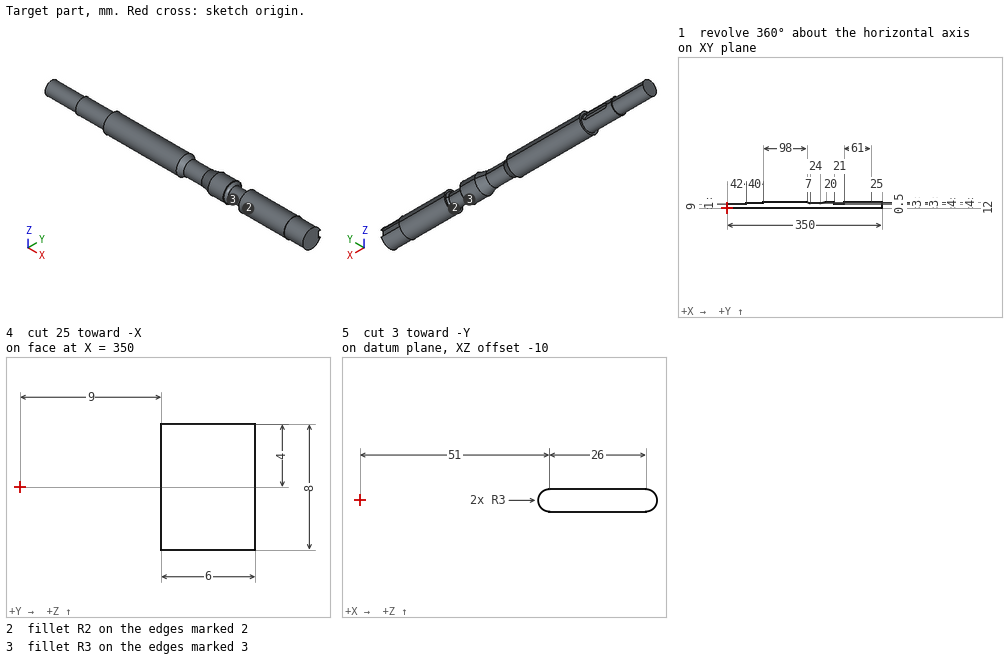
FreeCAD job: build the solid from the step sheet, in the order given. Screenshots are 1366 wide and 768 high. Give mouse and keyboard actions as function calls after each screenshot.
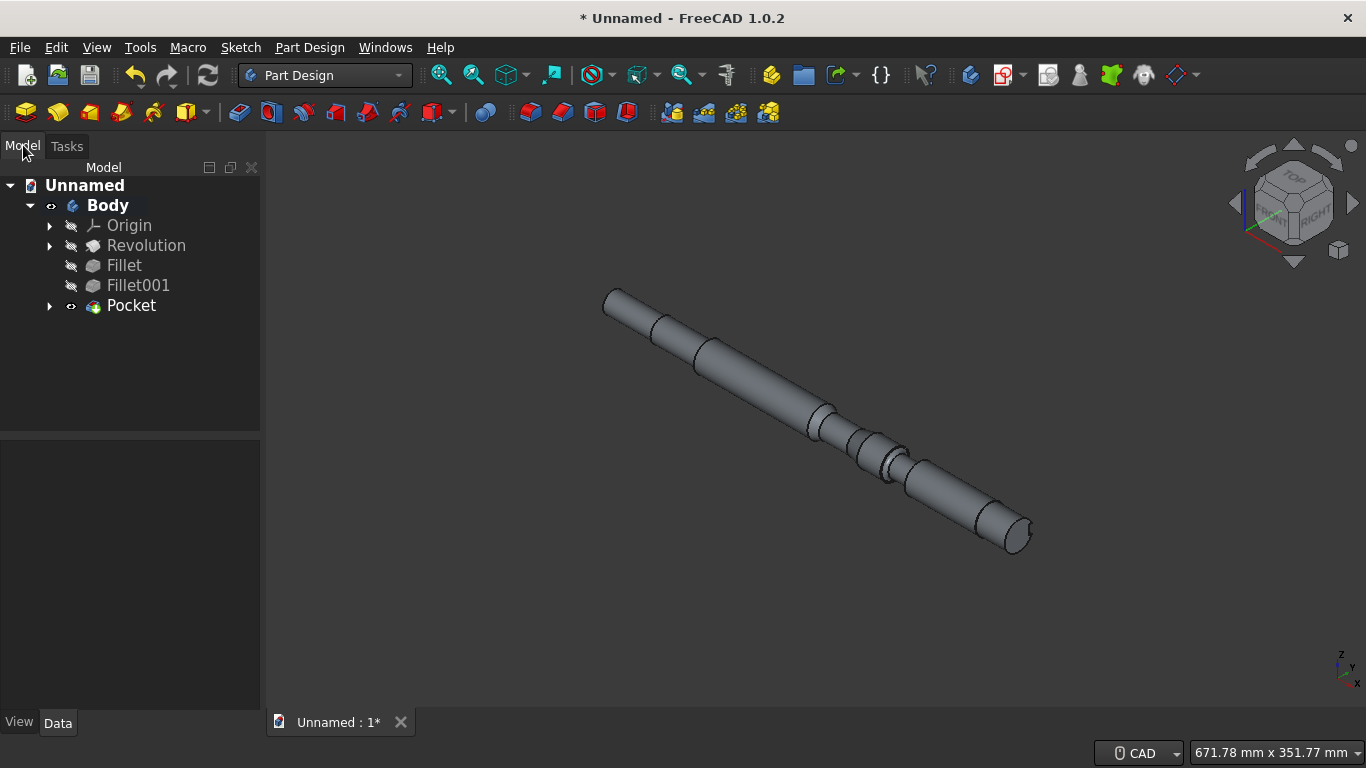
click(50, 226)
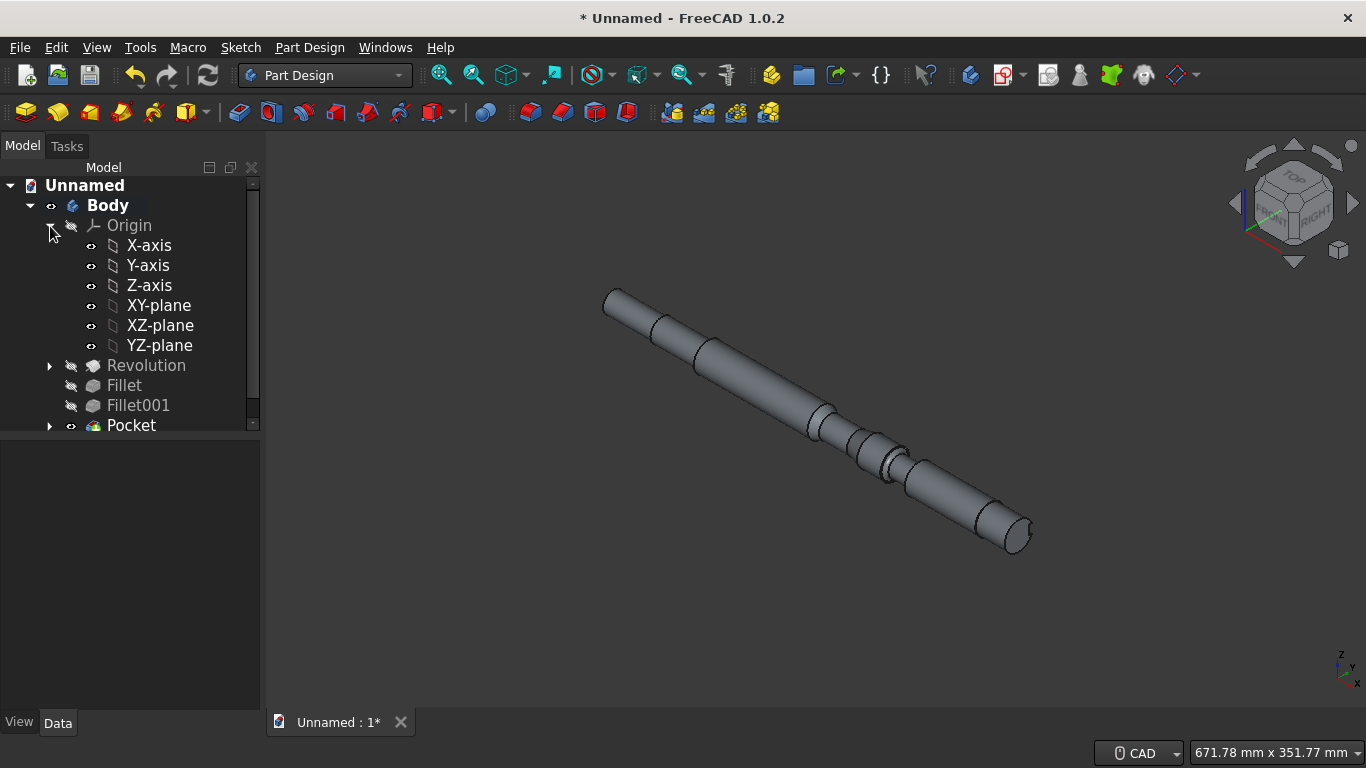
click(136, 326)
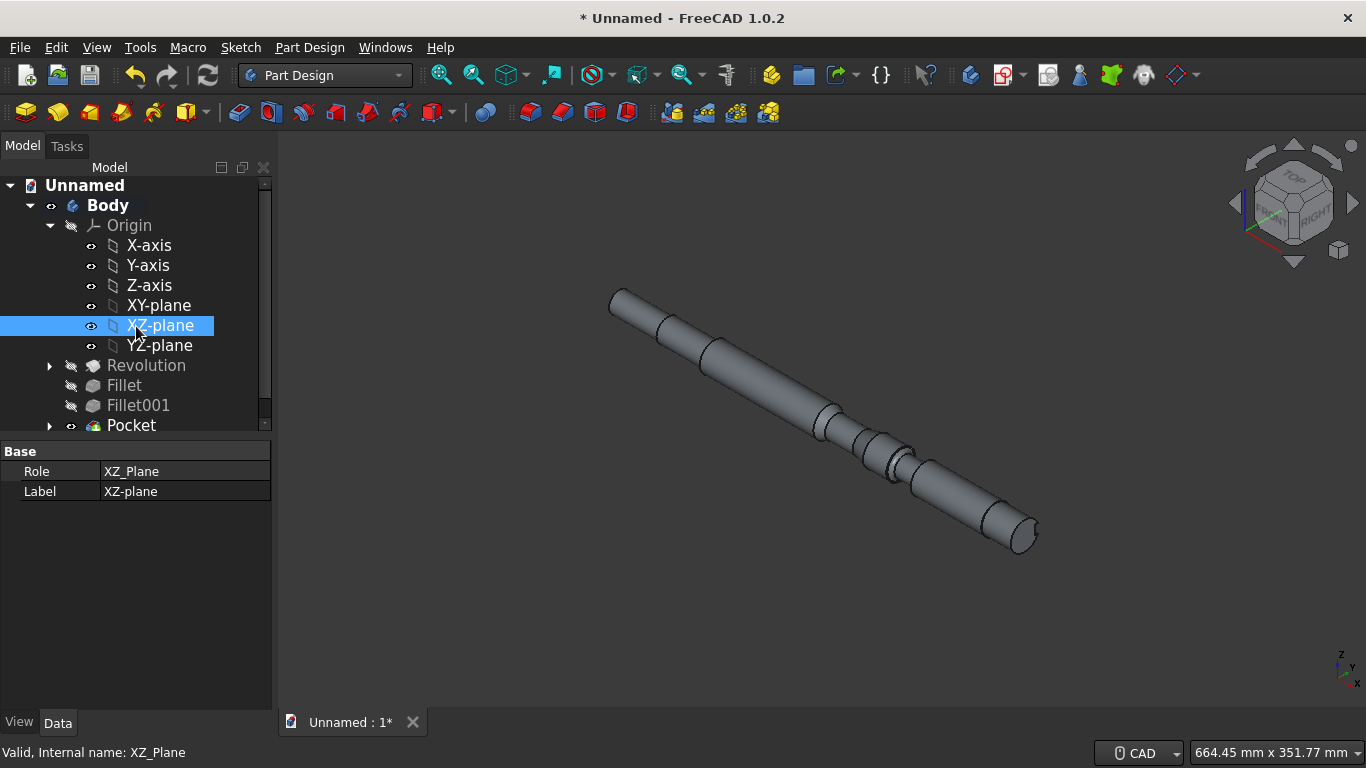
click(1176, 76)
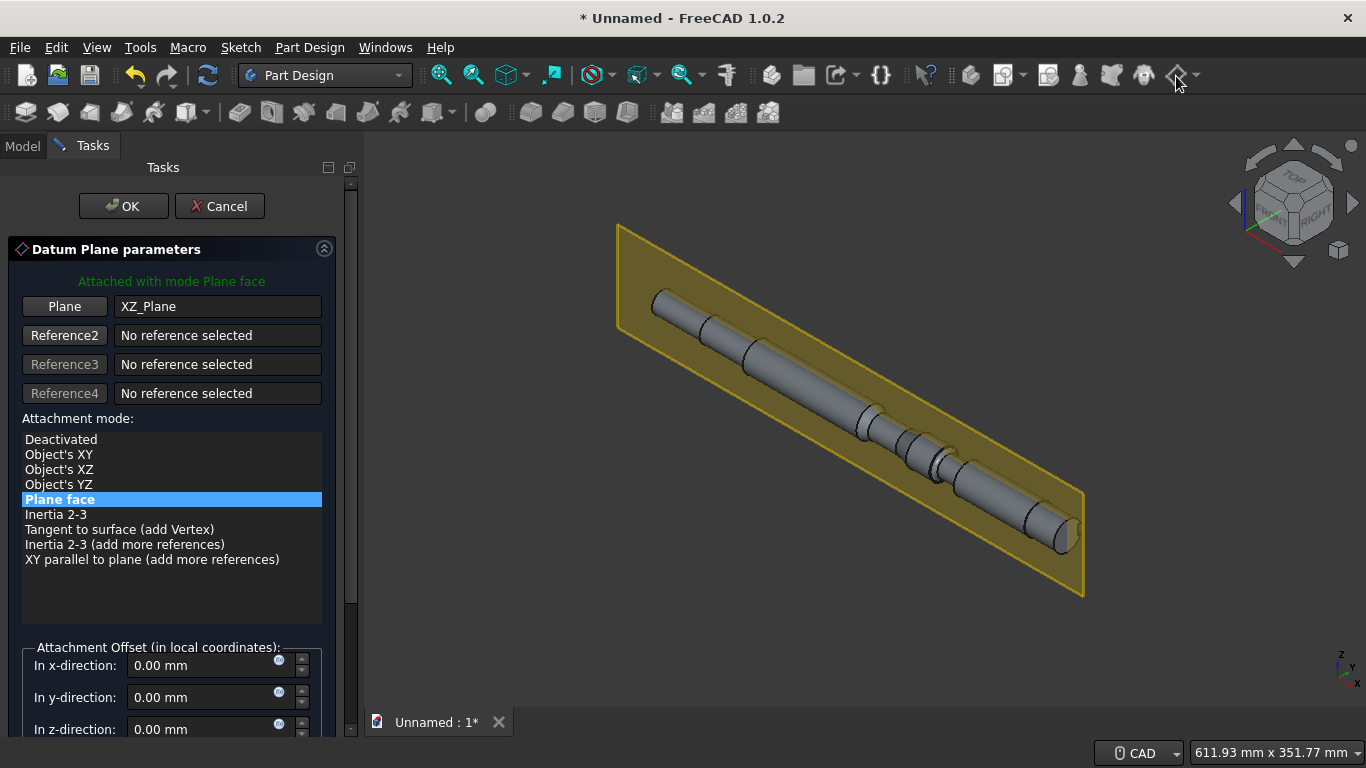
scroll(351, 456, down, 2)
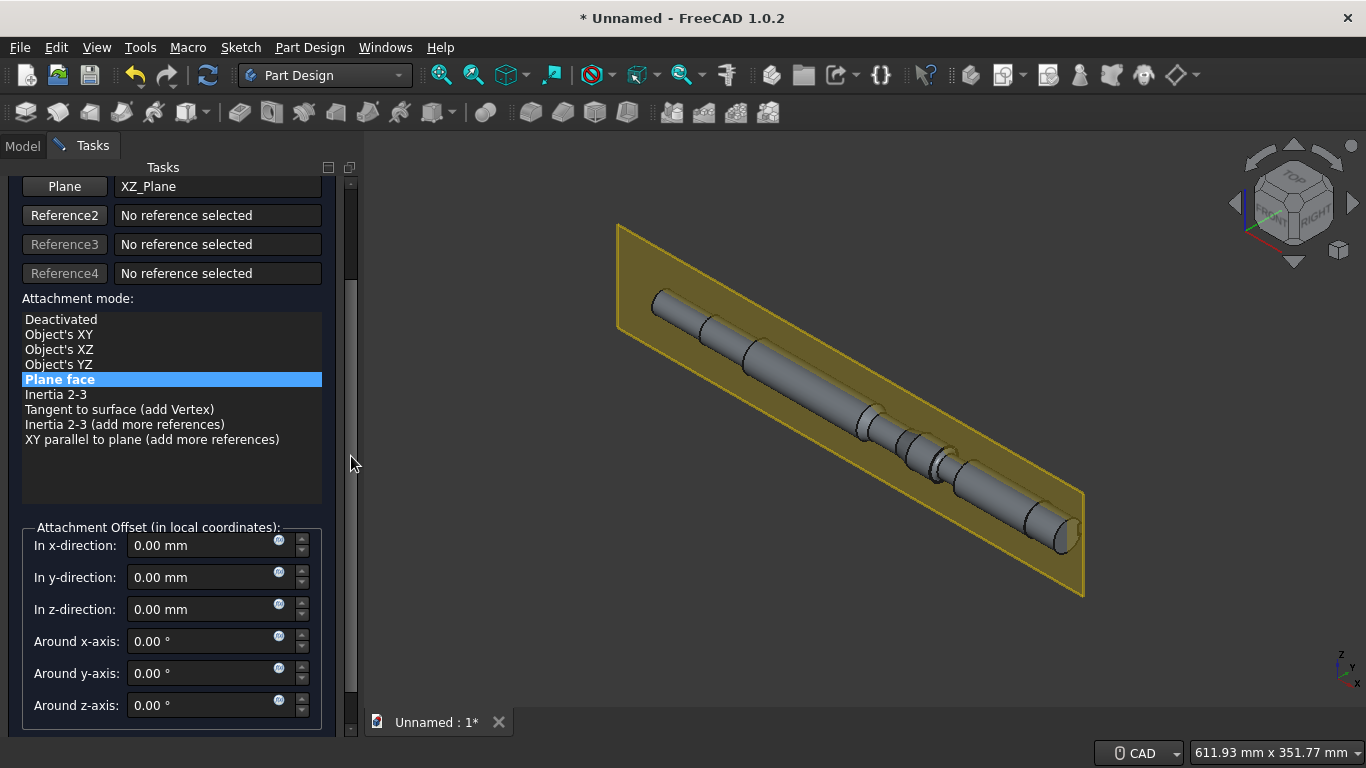
triple_click(210, 609)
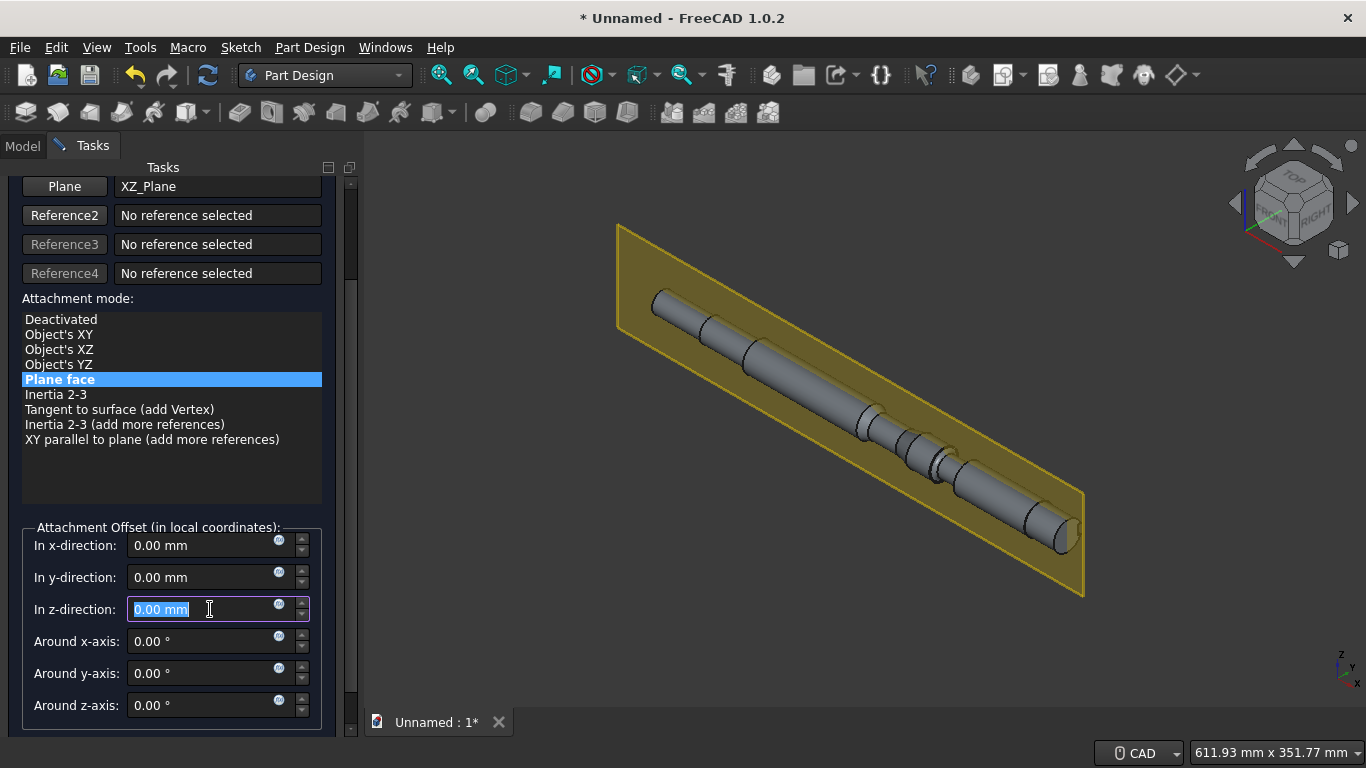
text(-10)
key(Tab)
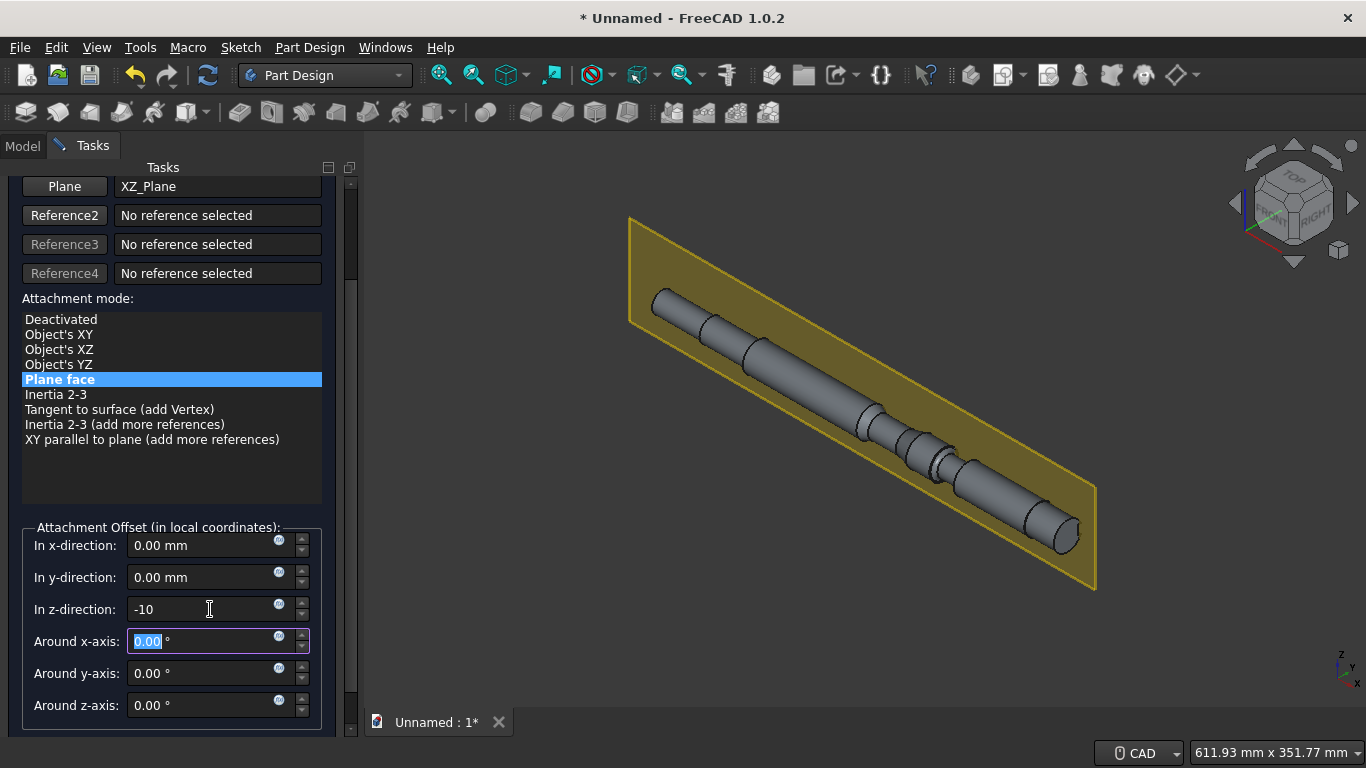
scroll(351, 456, up, 3)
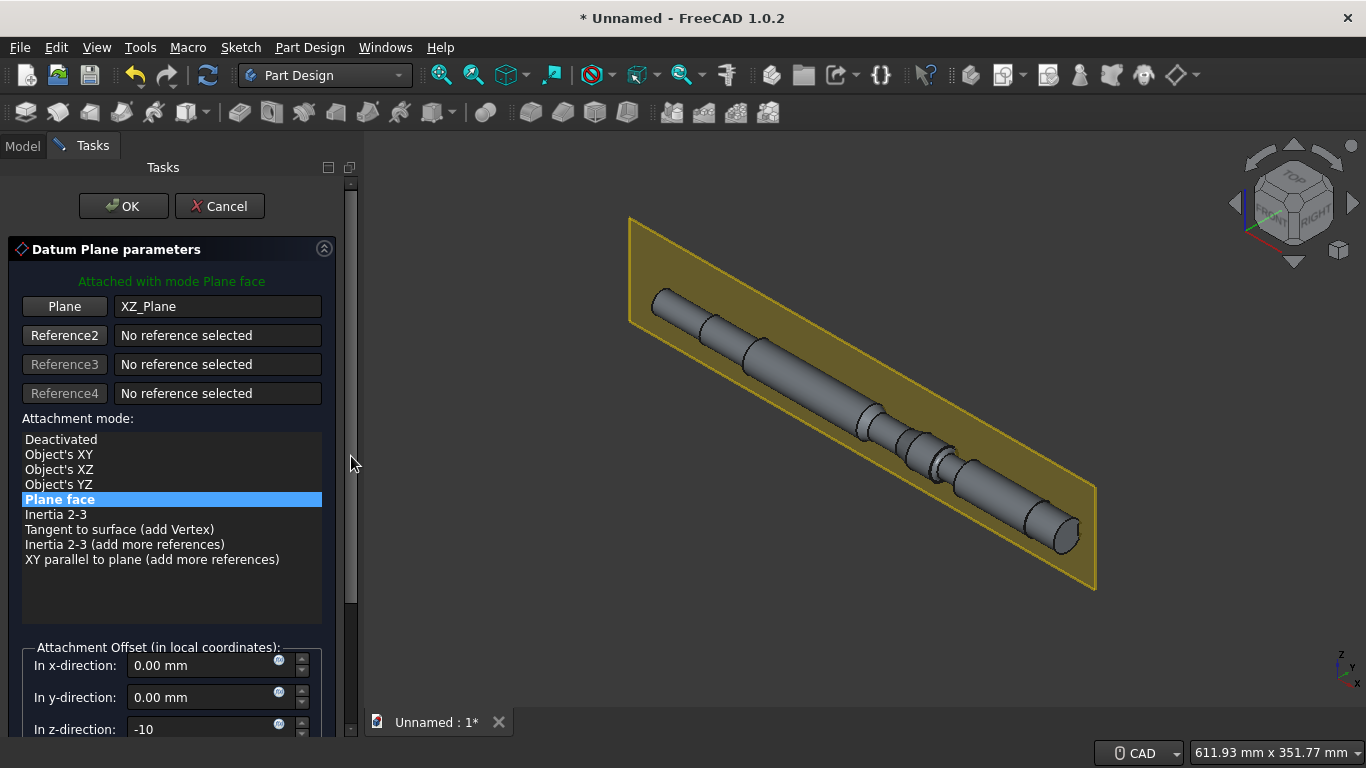
click(124, 206)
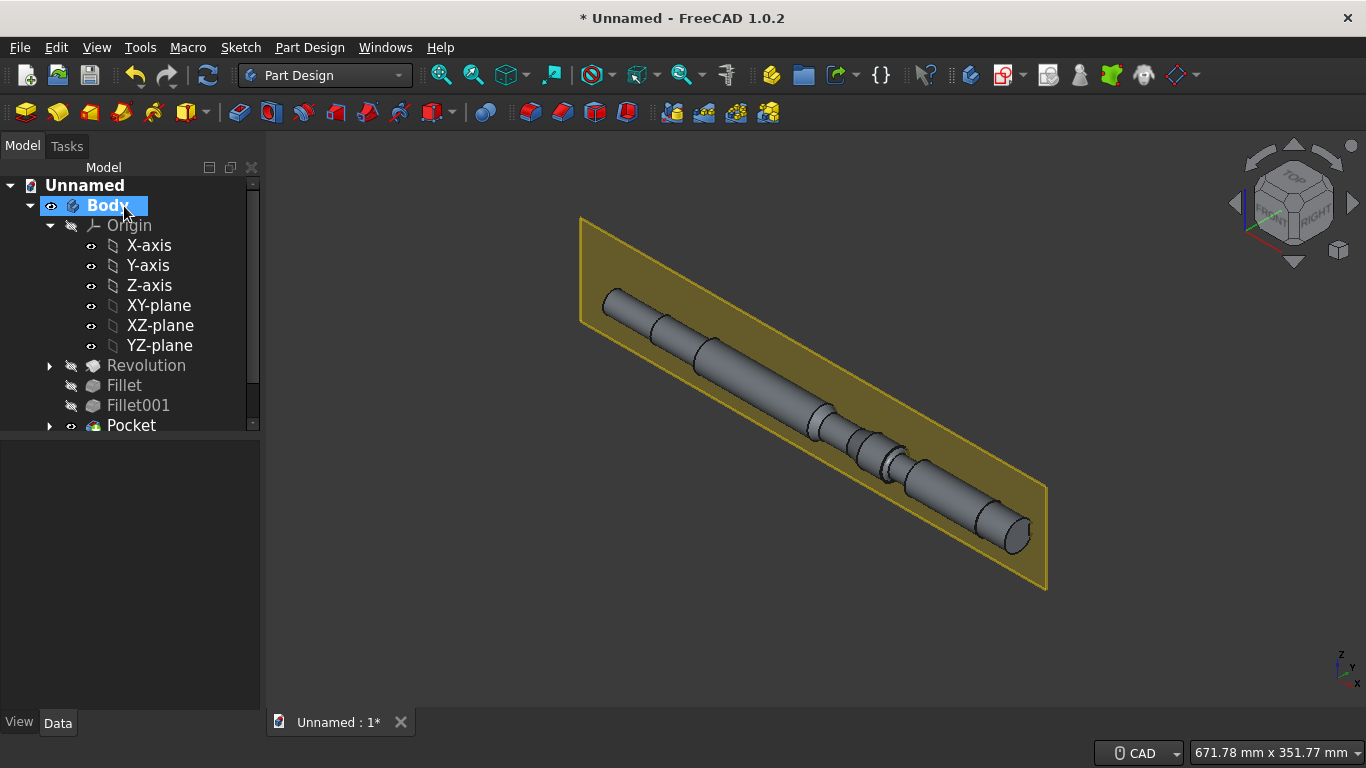
scroll(100, 301, down, 3)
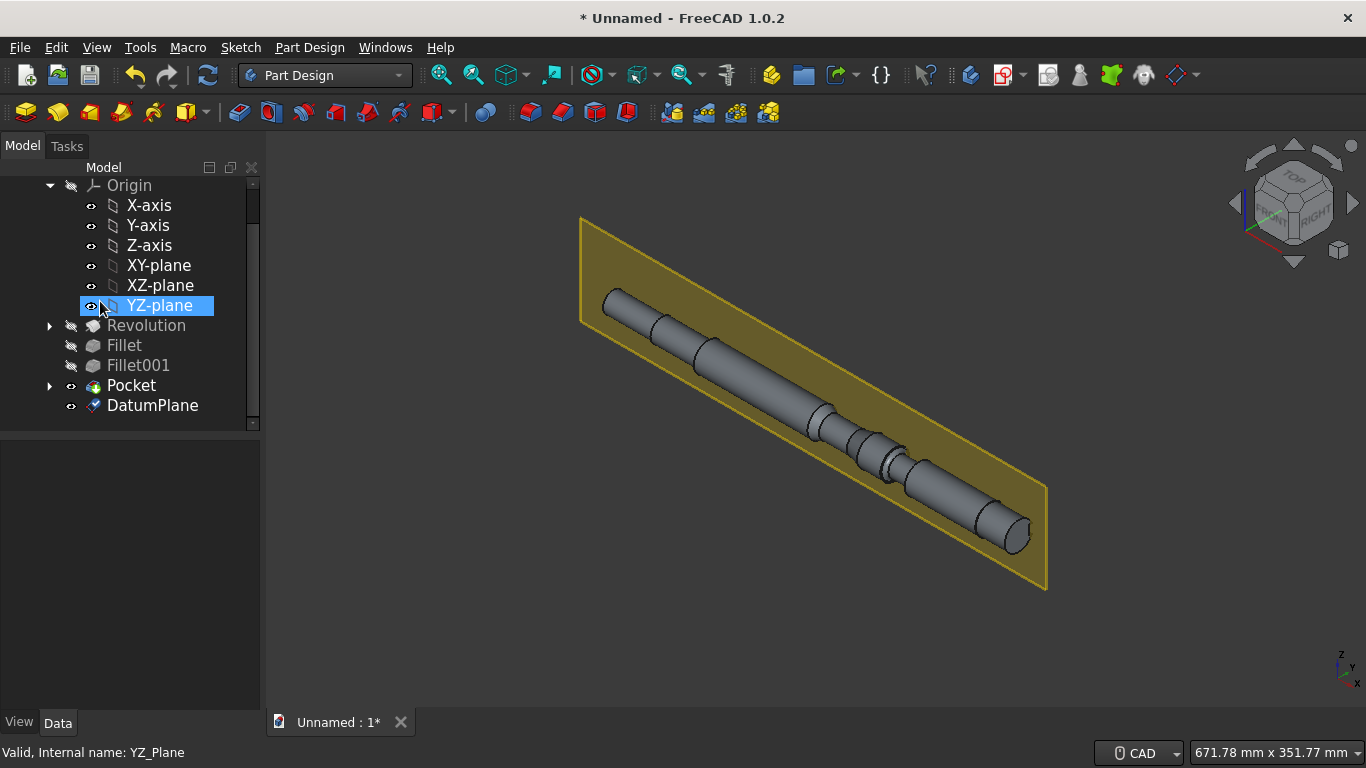
click(116, 406)